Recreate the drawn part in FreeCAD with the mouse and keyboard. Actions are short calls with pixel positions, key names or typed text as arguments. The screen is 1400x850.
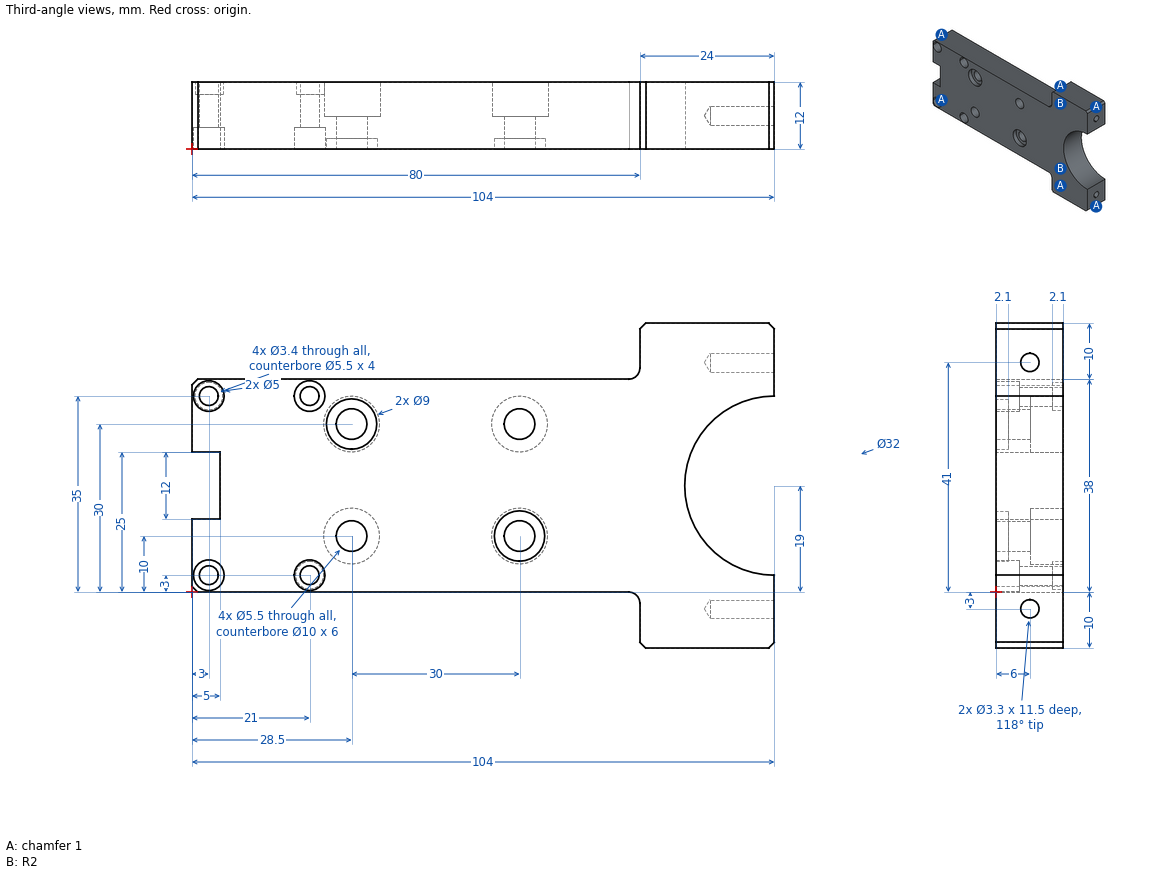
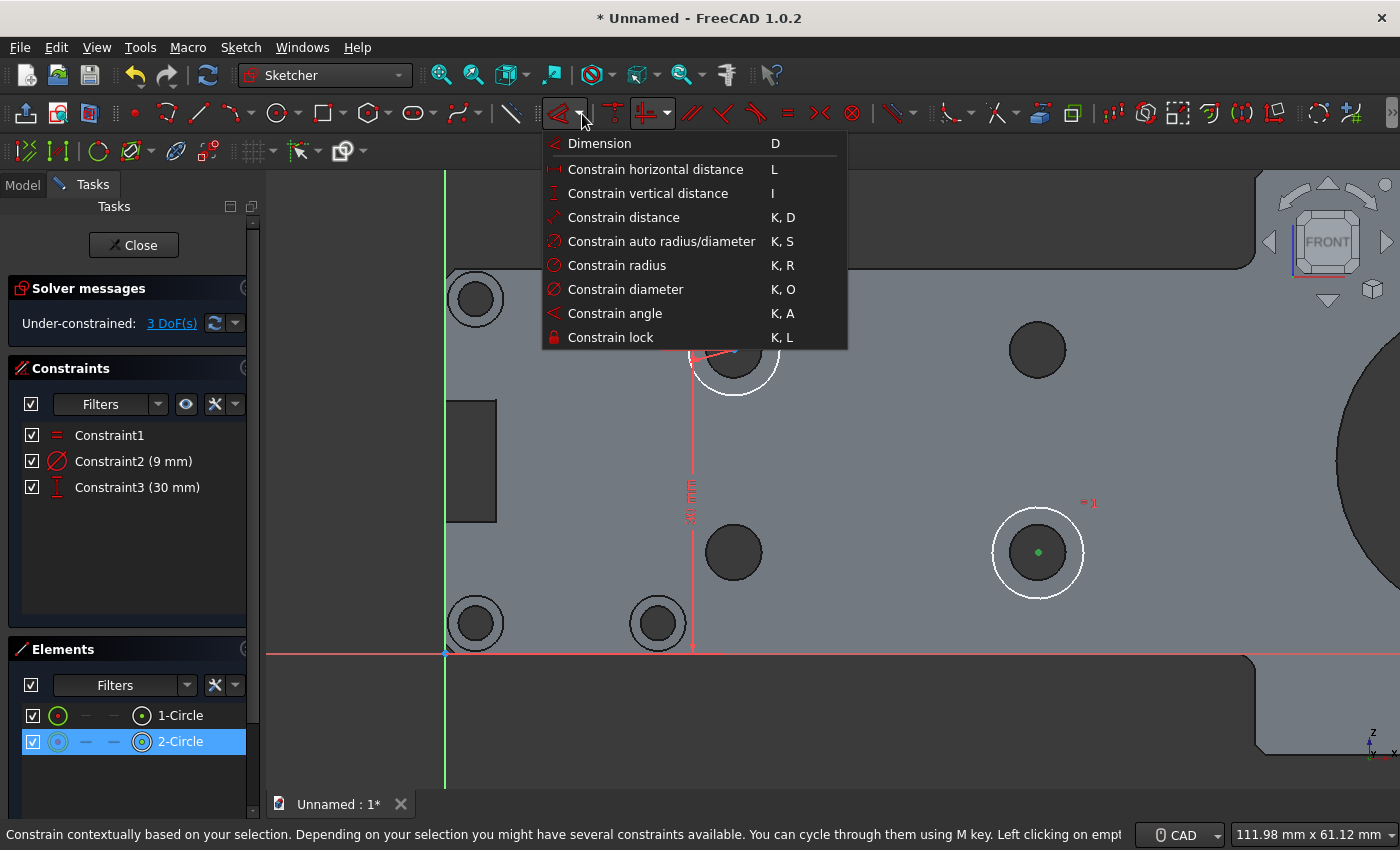
click(695, 193)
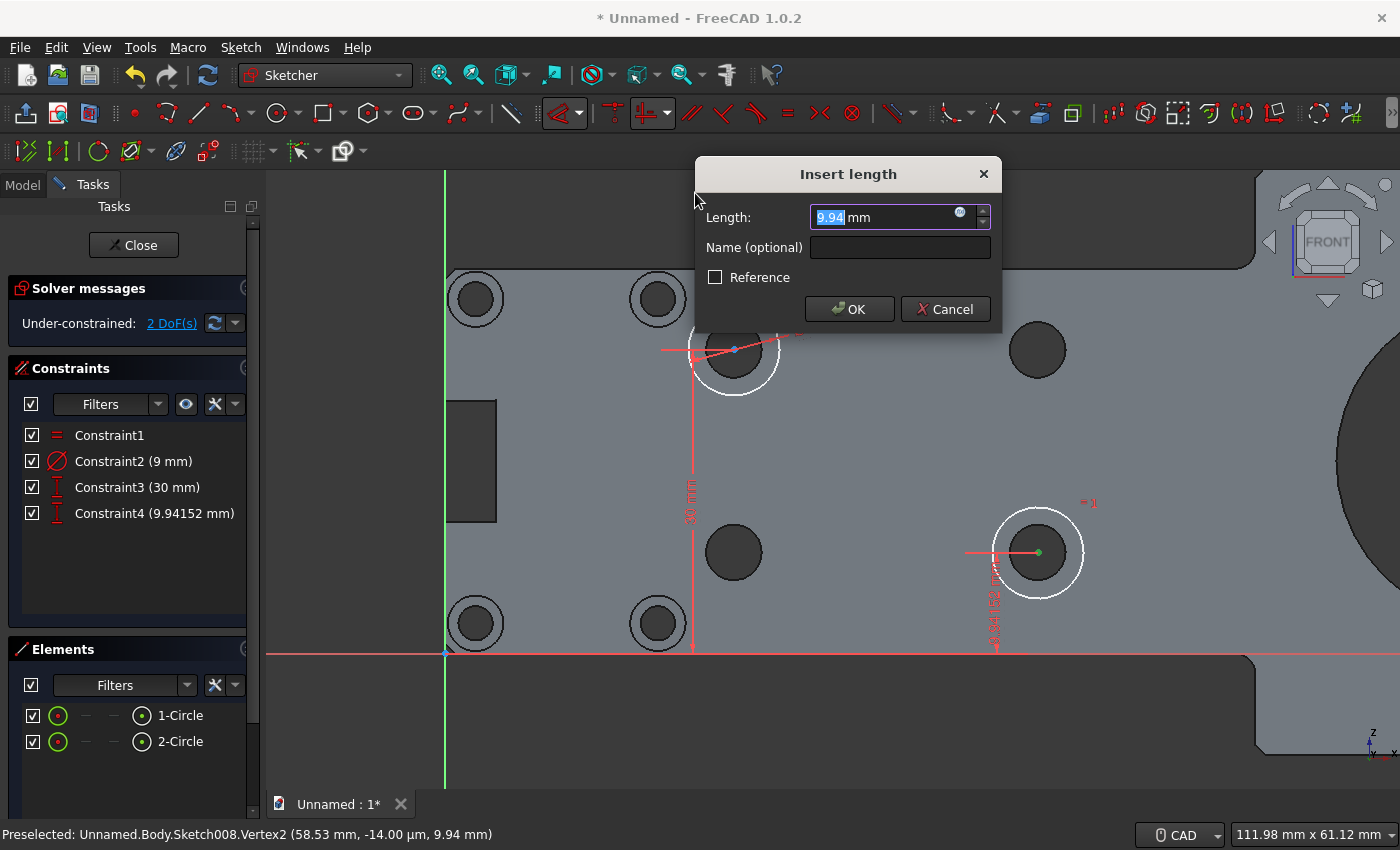
text(10)
key(Return)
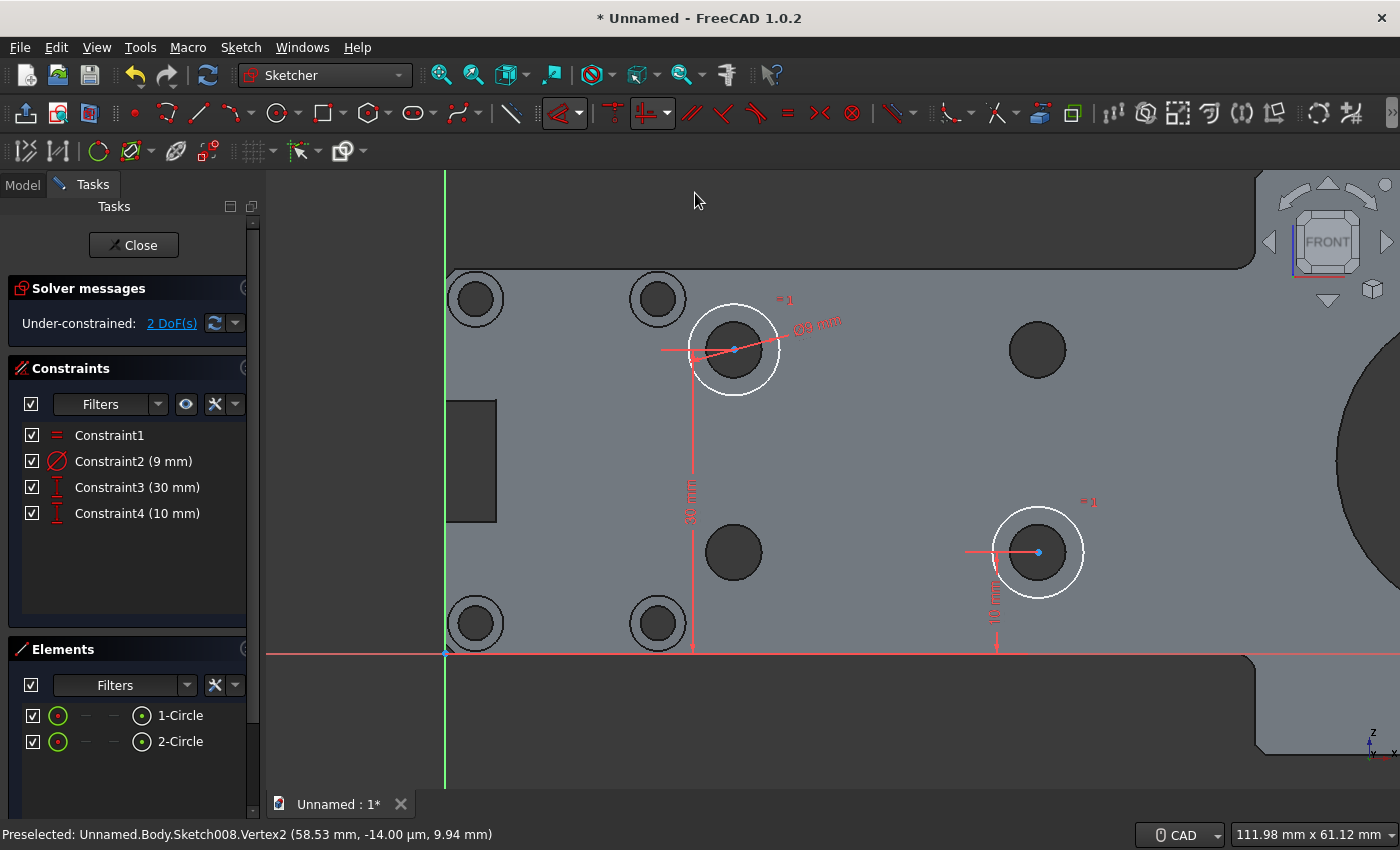
click(734, 350)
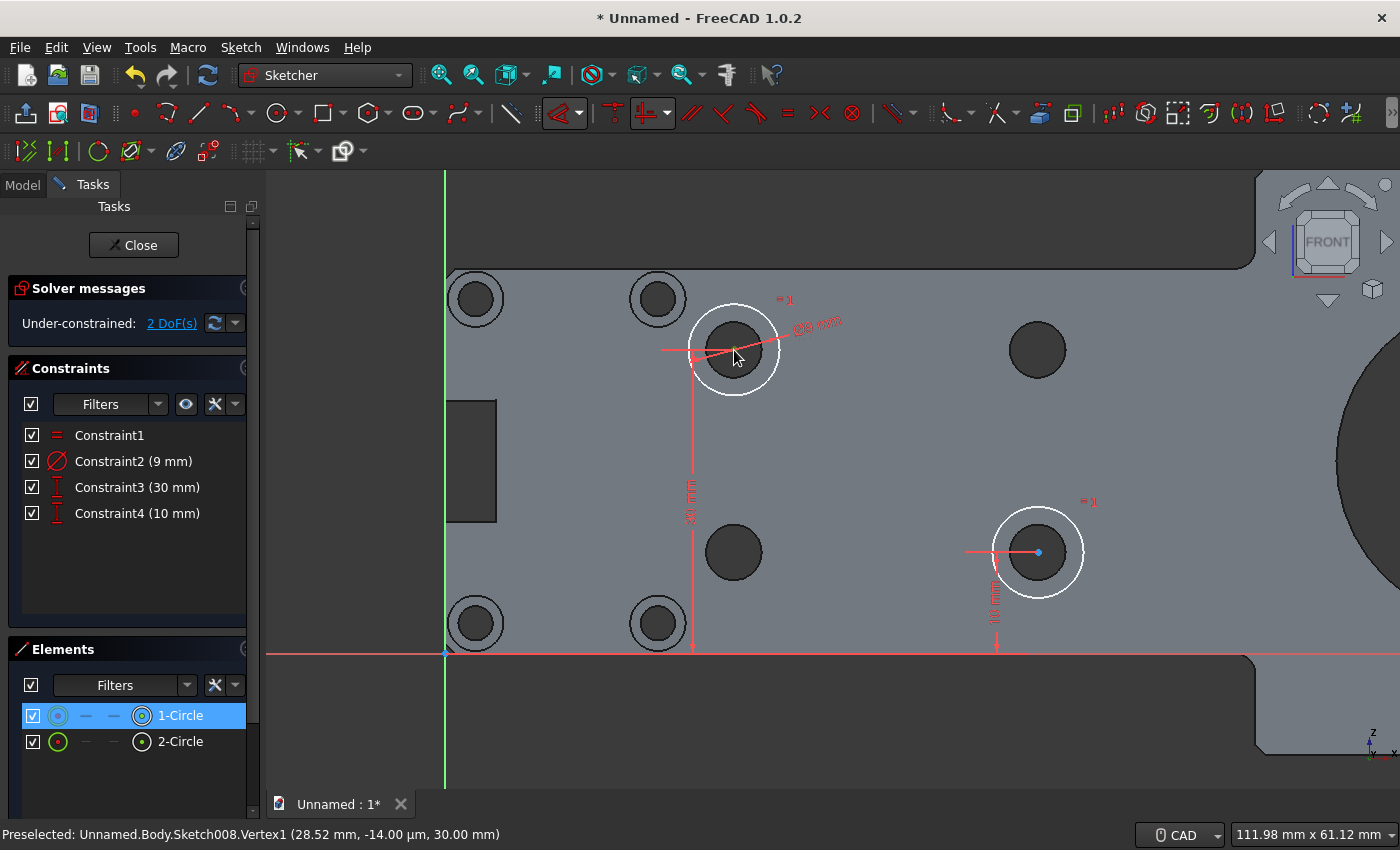
click(1038, 552)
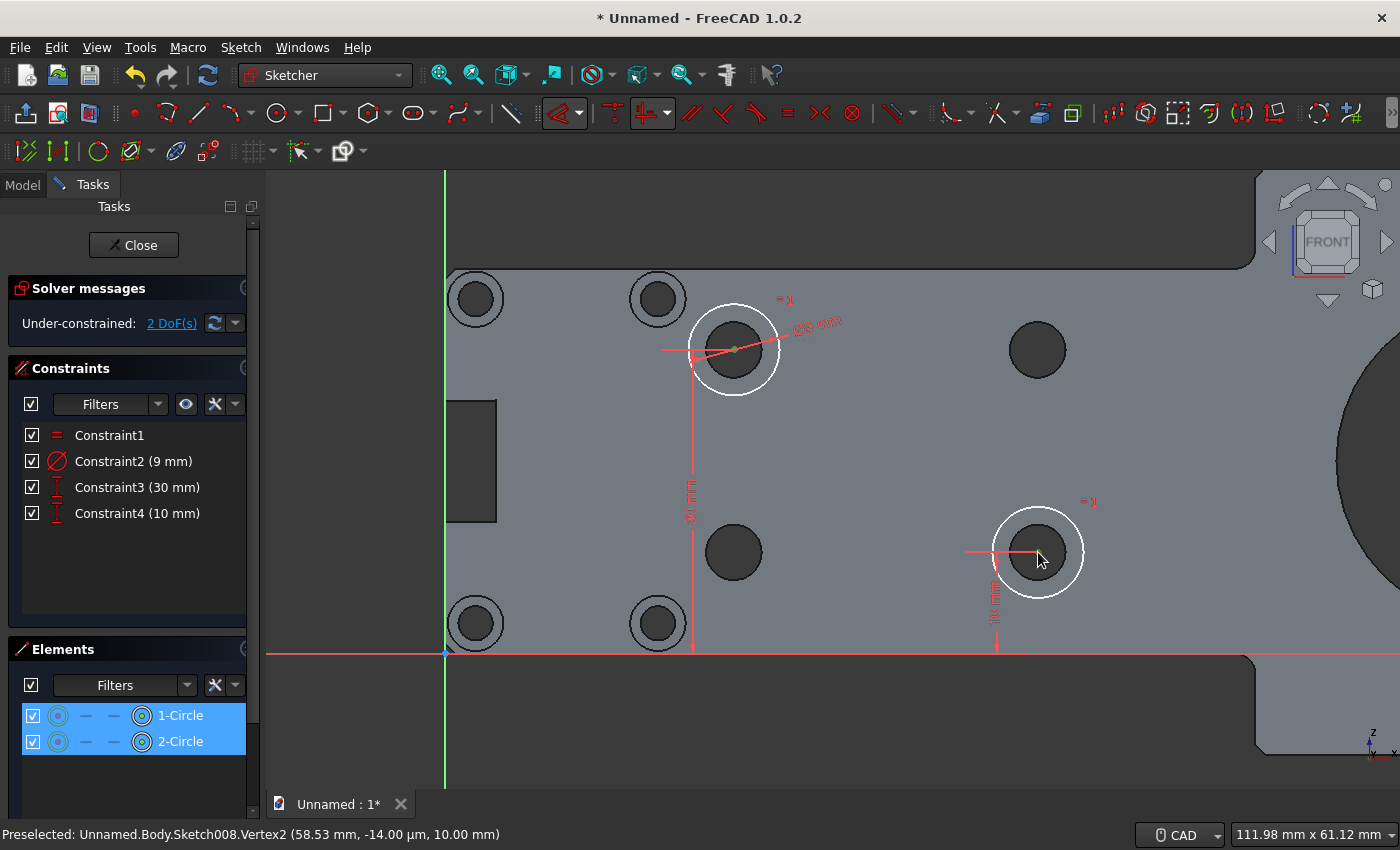
click(582, 114)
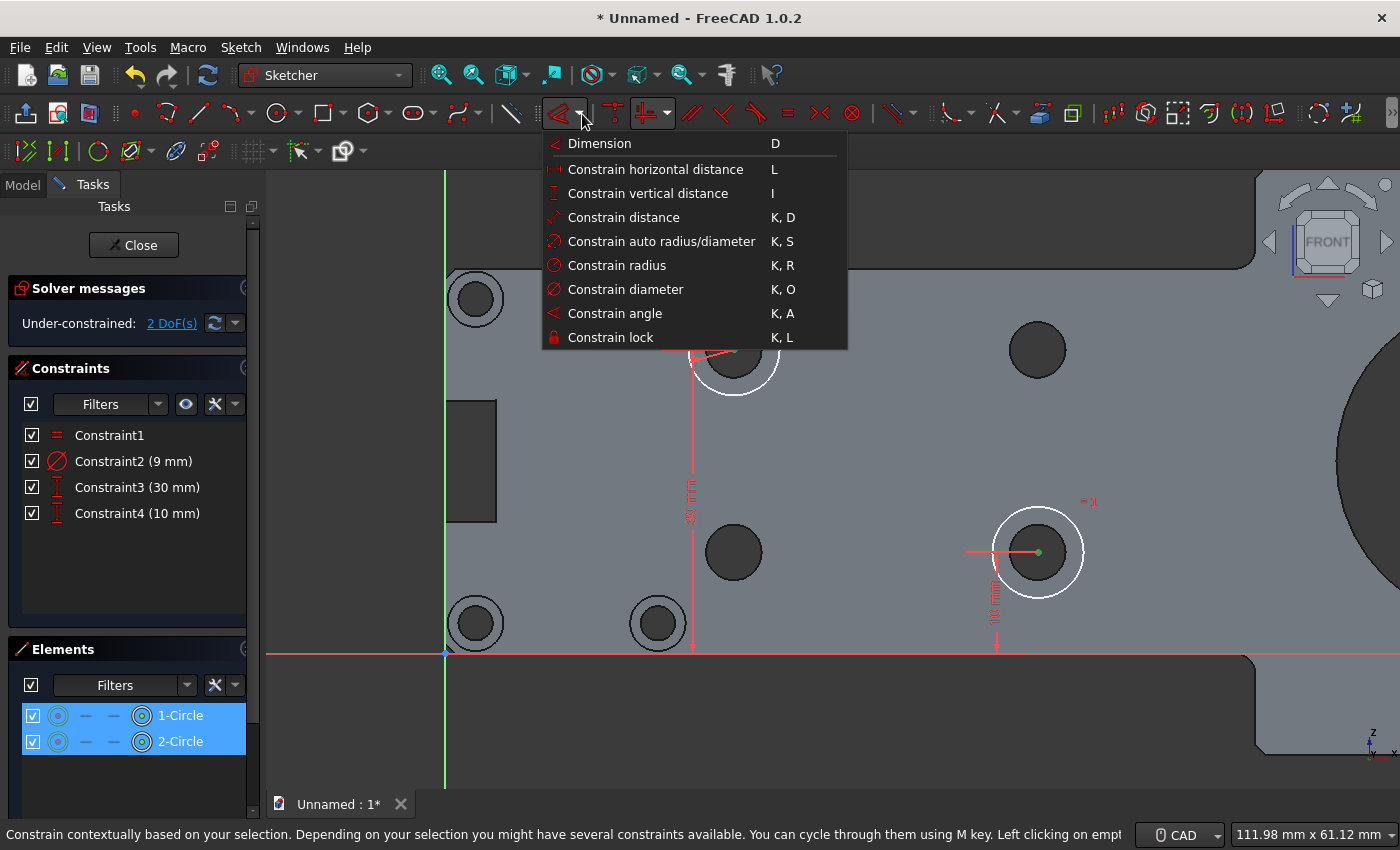
click(695, 169)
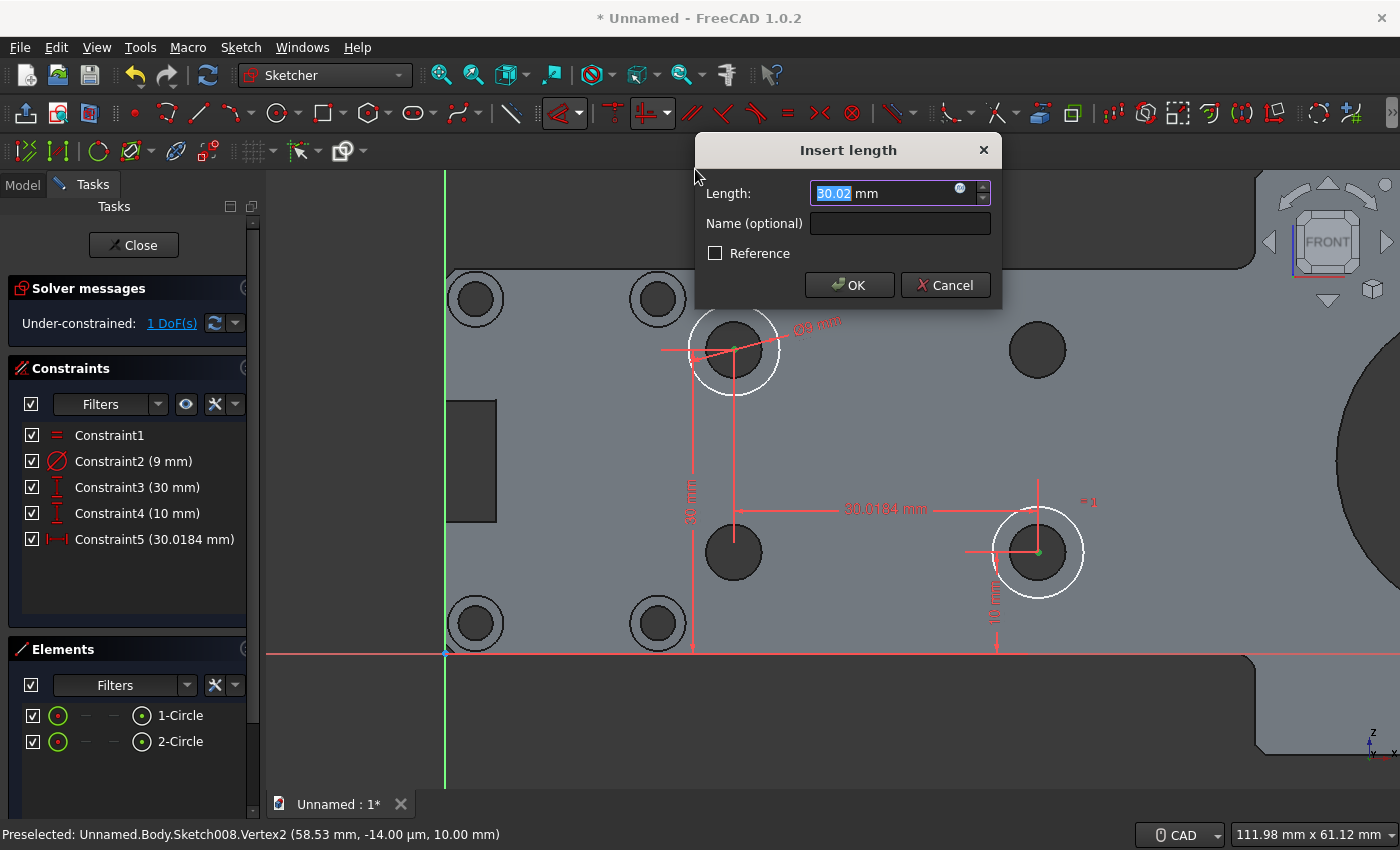
text(30)
key(Return)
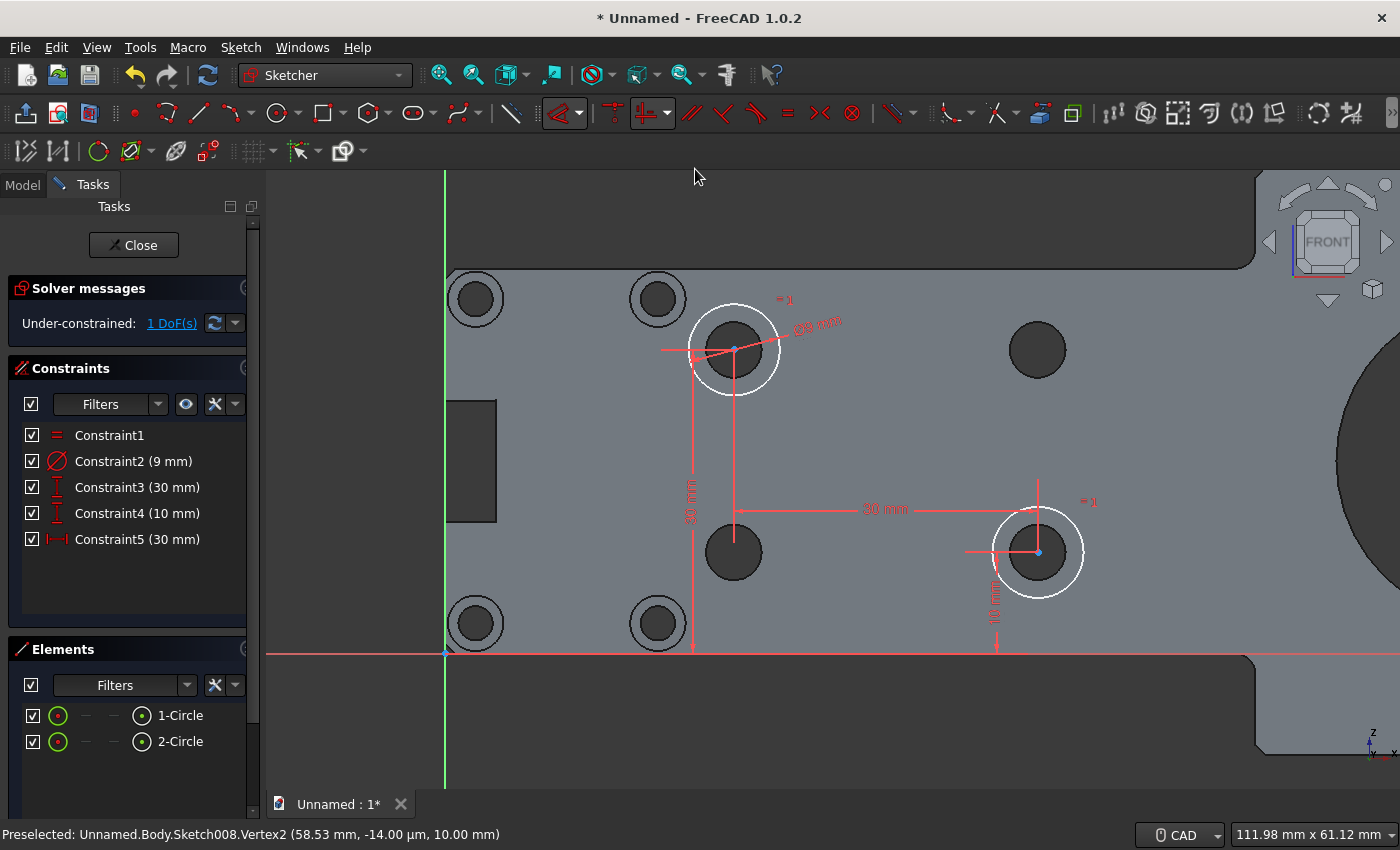
click(734, 350)